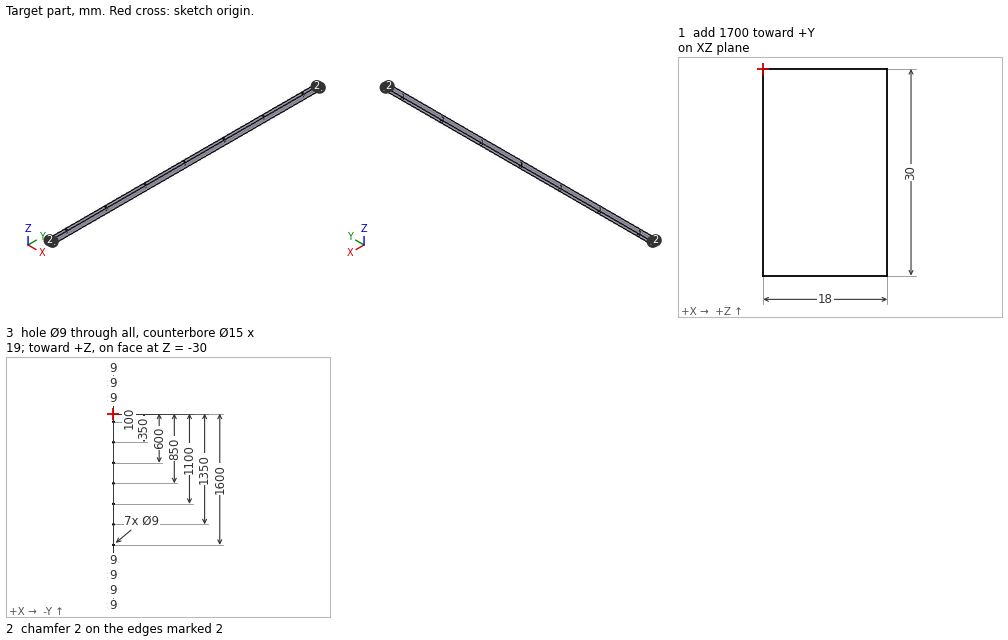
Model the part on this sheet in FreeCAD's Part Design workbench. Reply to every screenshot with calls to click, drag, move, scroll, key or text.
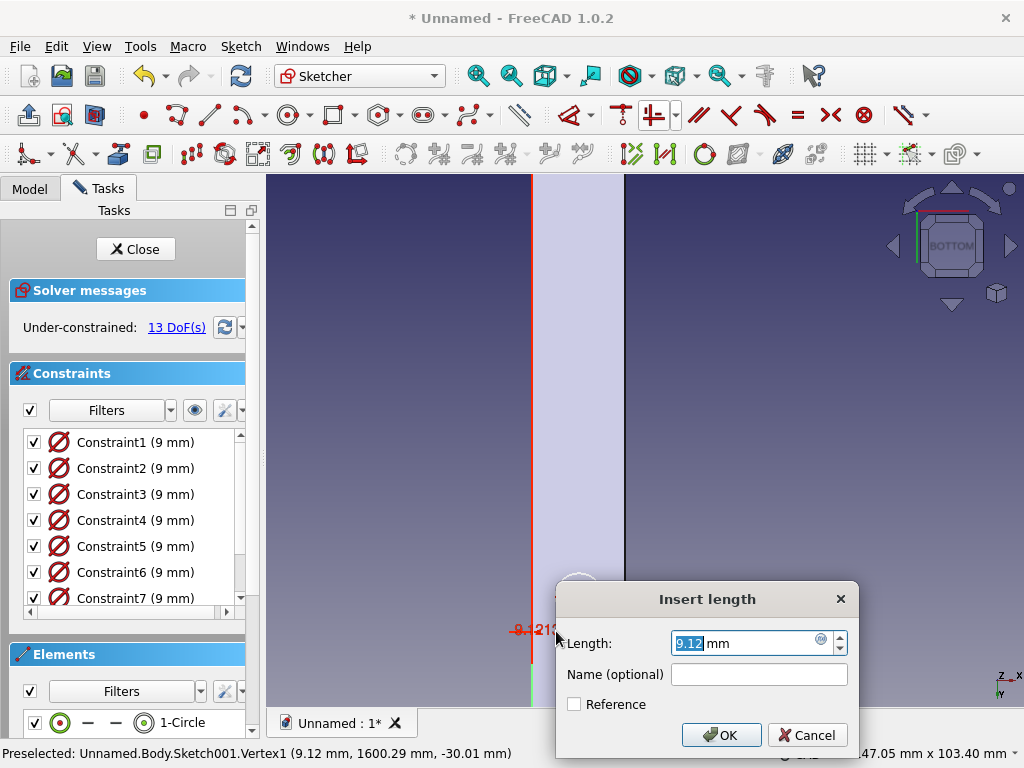
text(9)
key(Return)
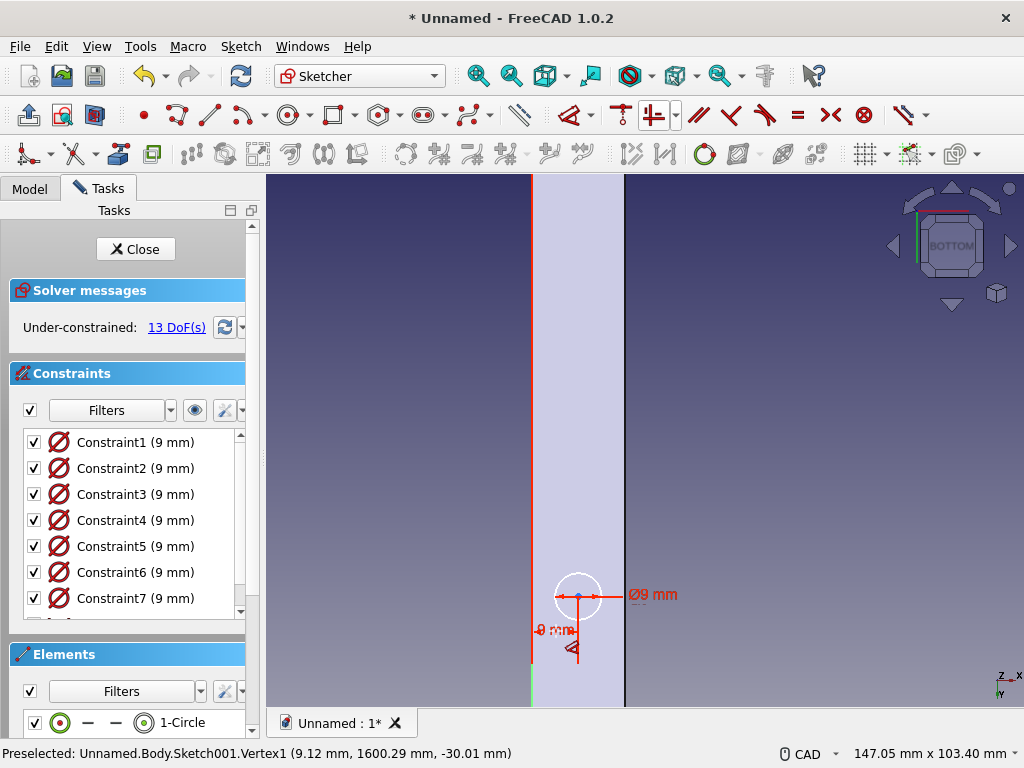
scroll(577, 648, down, 15)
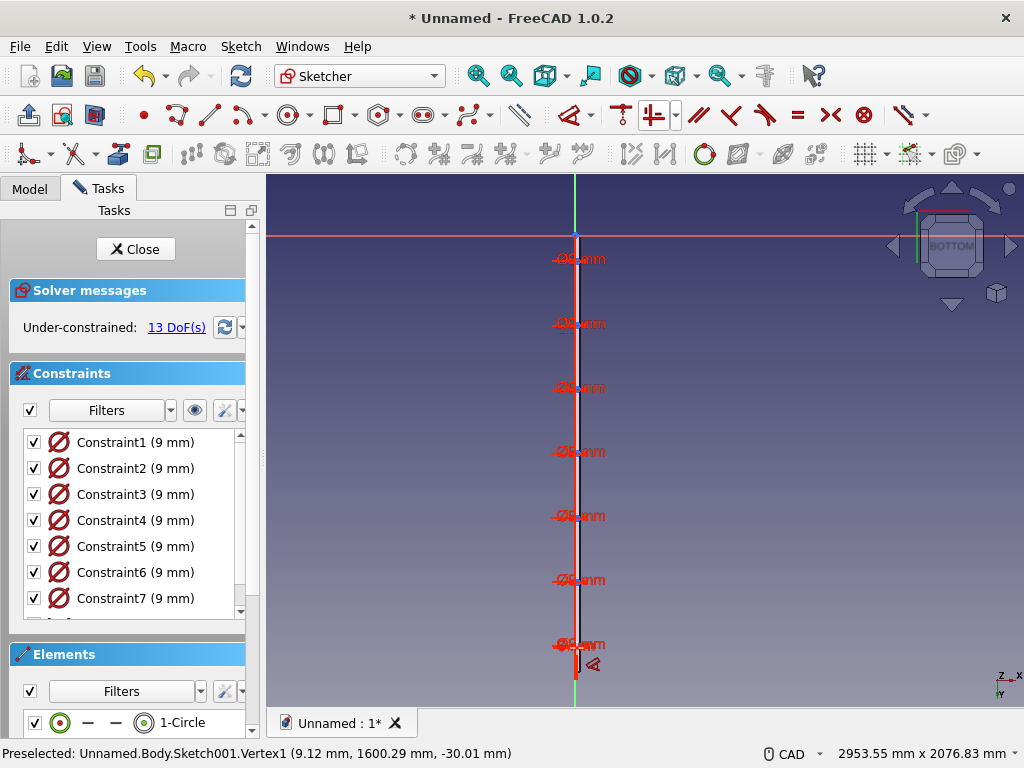
scroll(577, 582, up, 15)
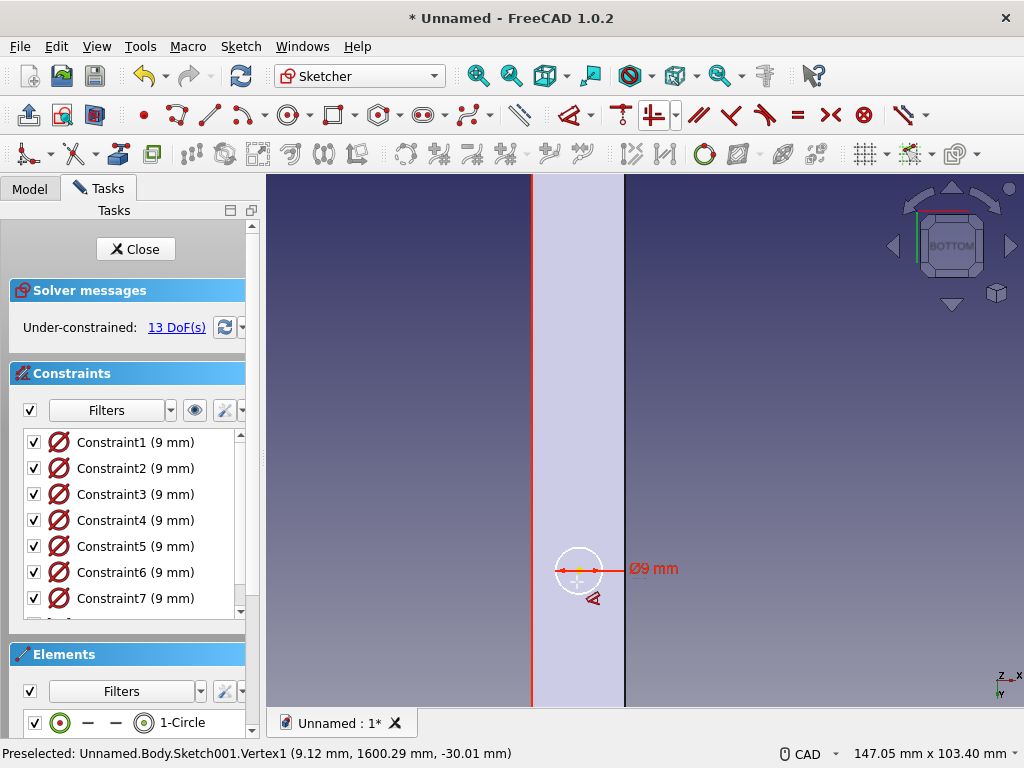
click(579, 571)
click(556, 605)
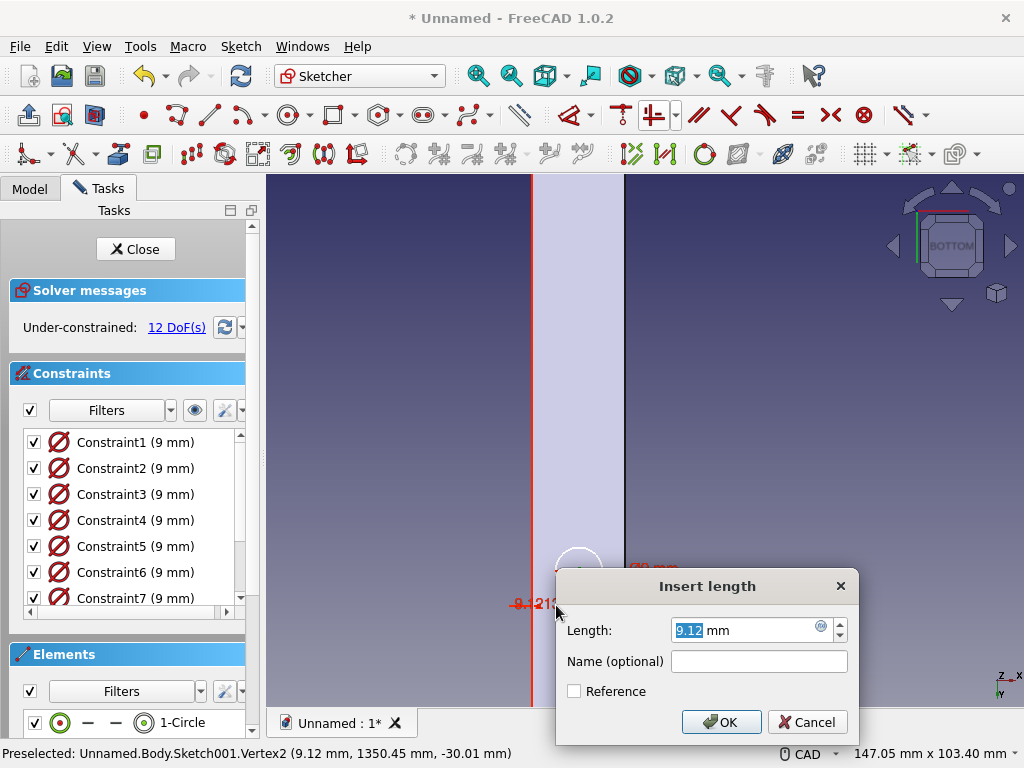
text(9)
key(Return)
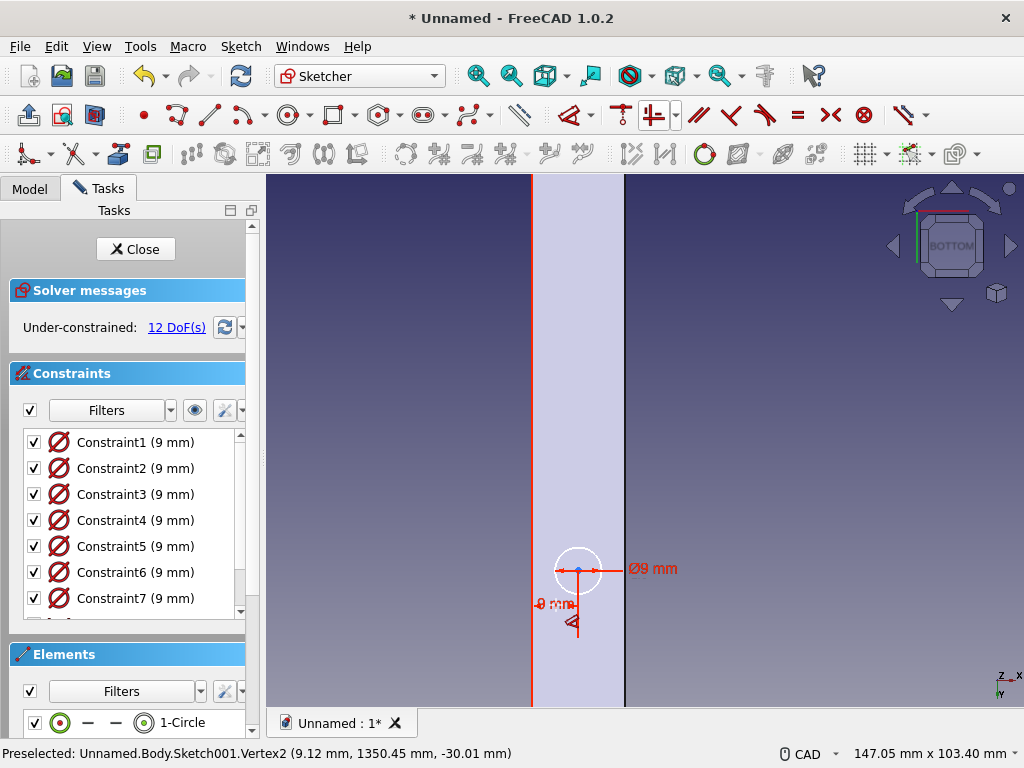
scroll(577, 582, down, 15)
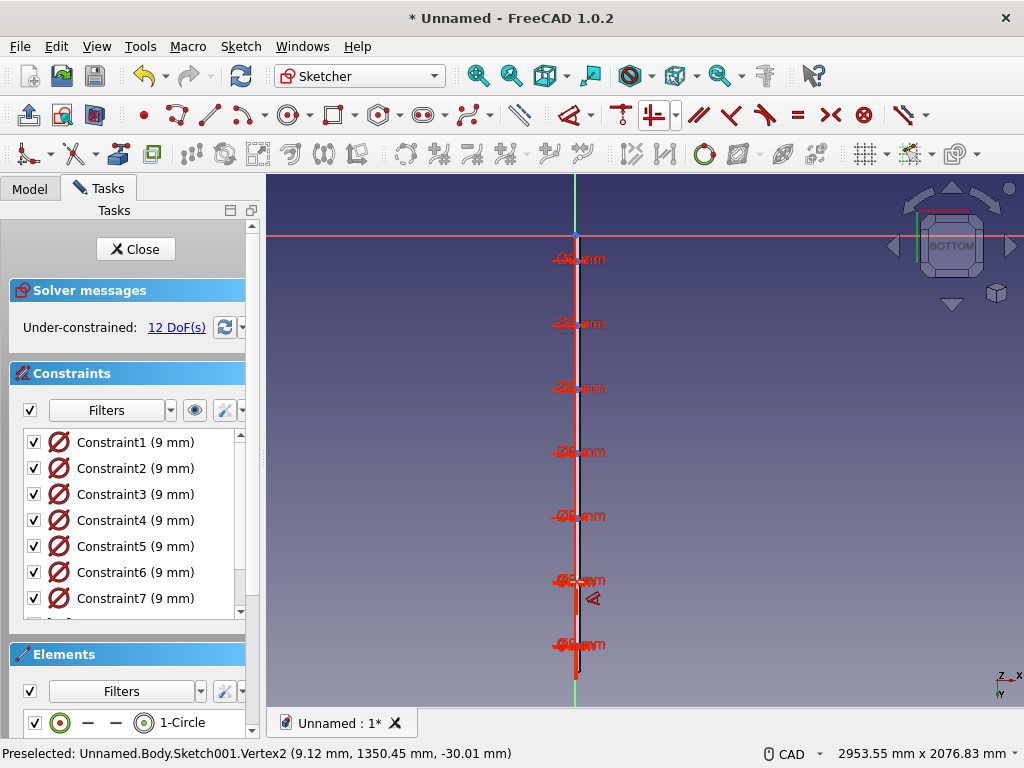
scroll(577, 518, up, 15)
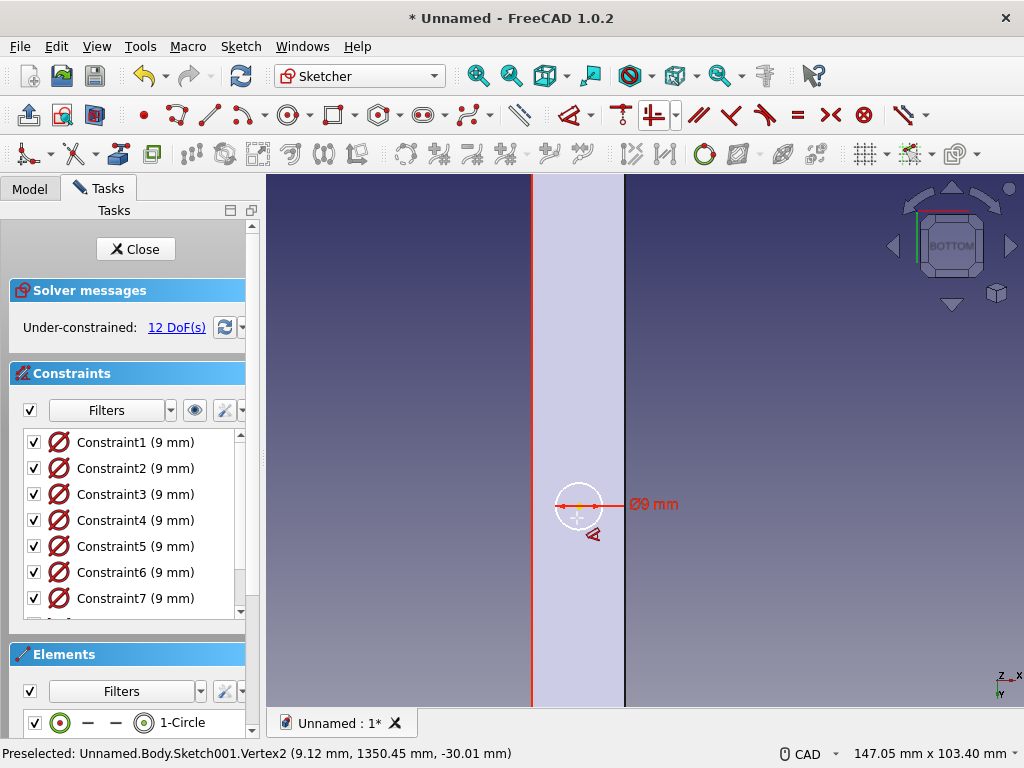
click(579, 506)
click(556, 540)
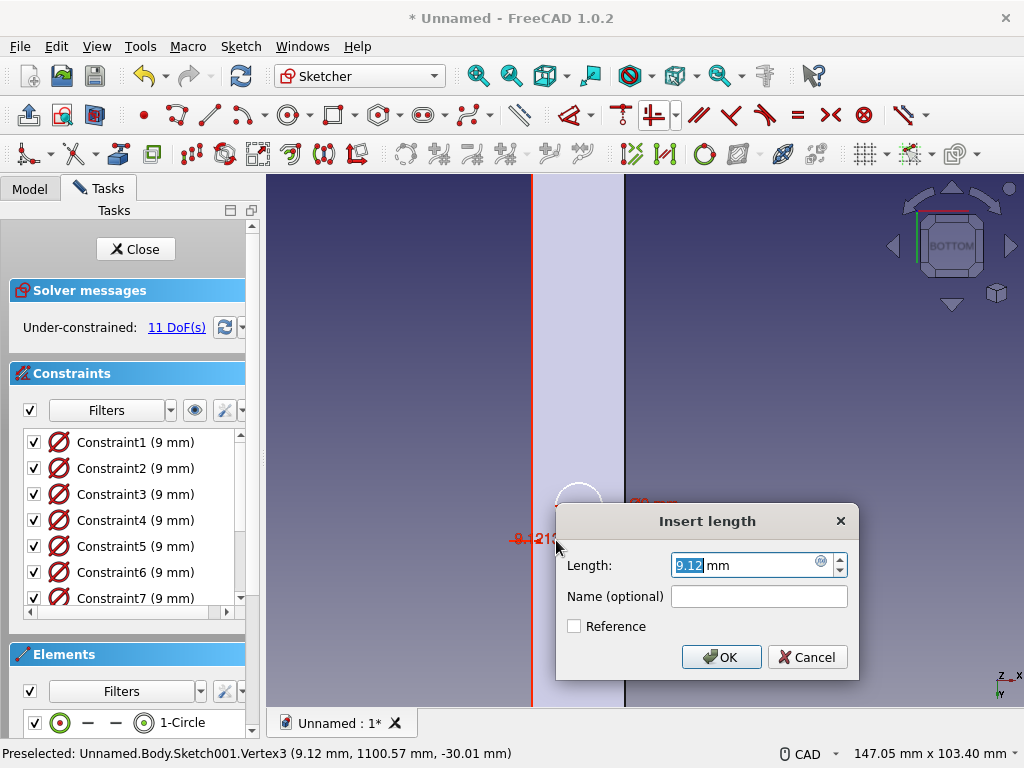
text(9)
key(Return)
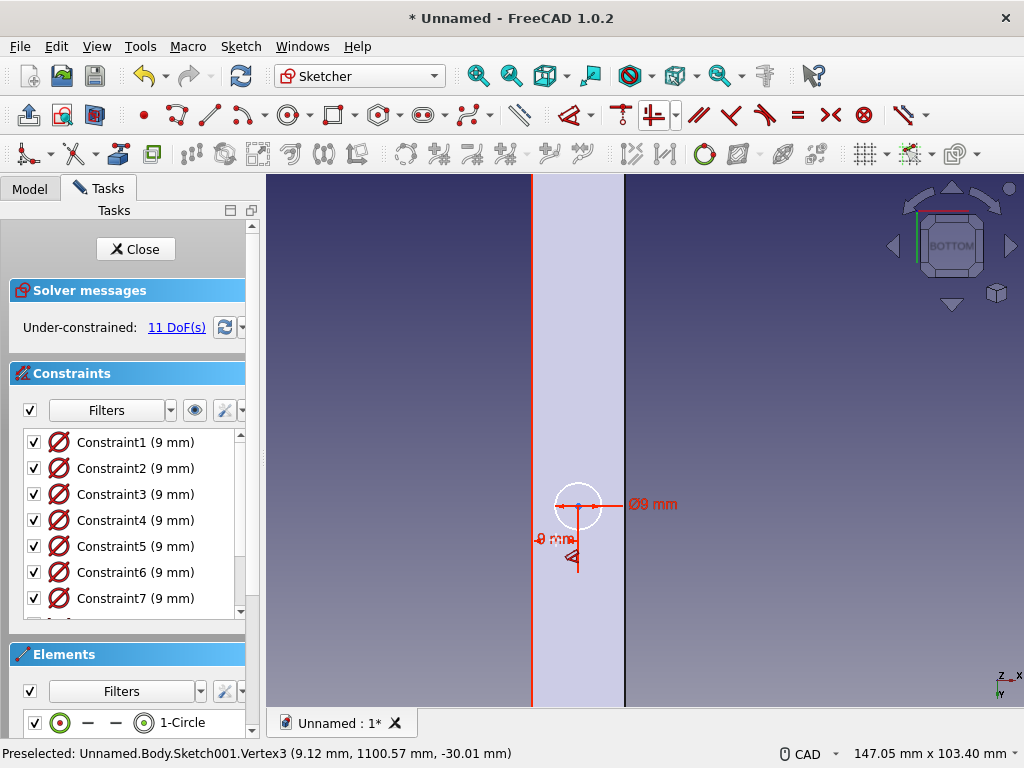
scroll(577, 518, down, 15)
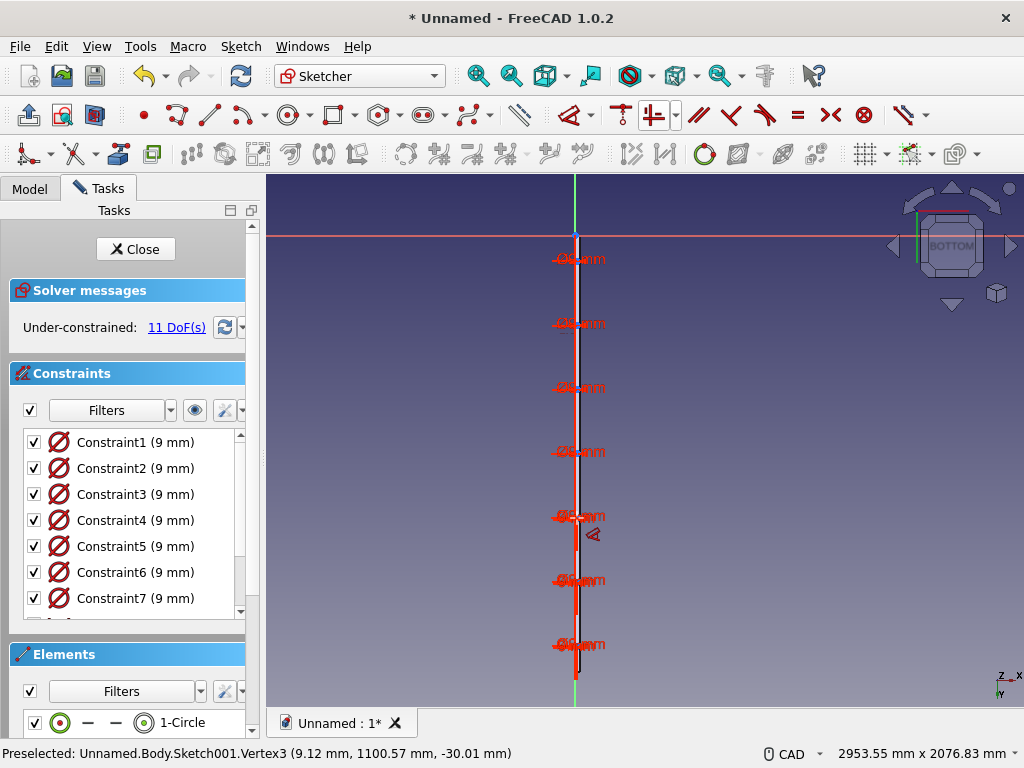
scroll(577, 390, up, 15)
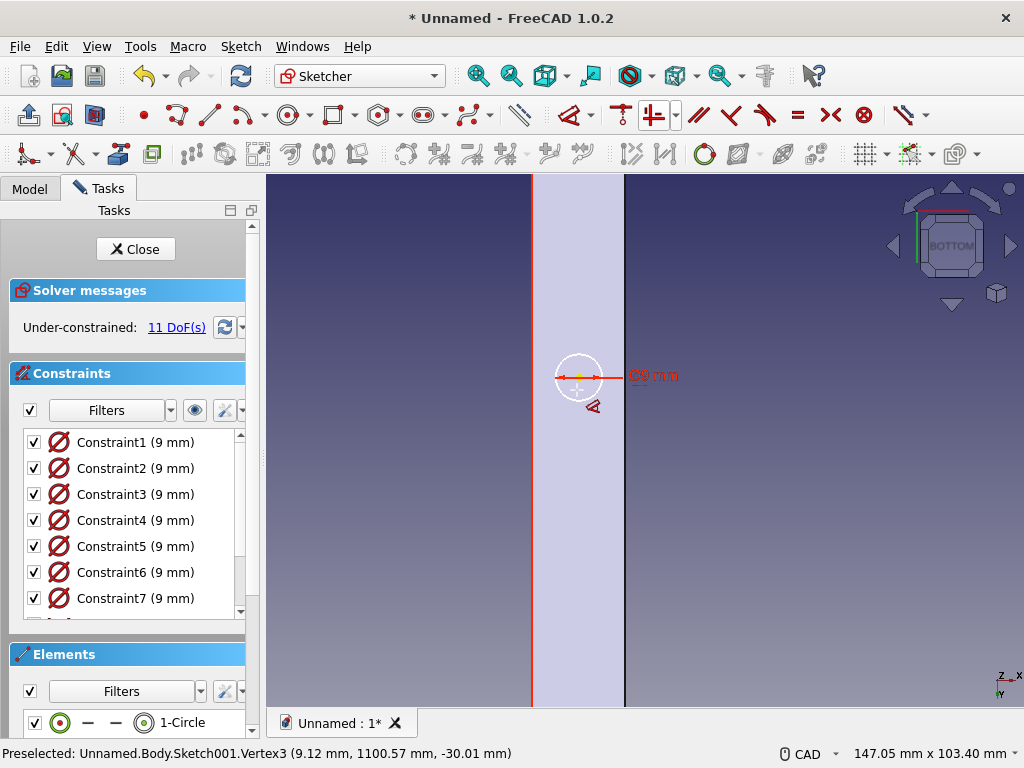
click(579, 378)
click(556, 412)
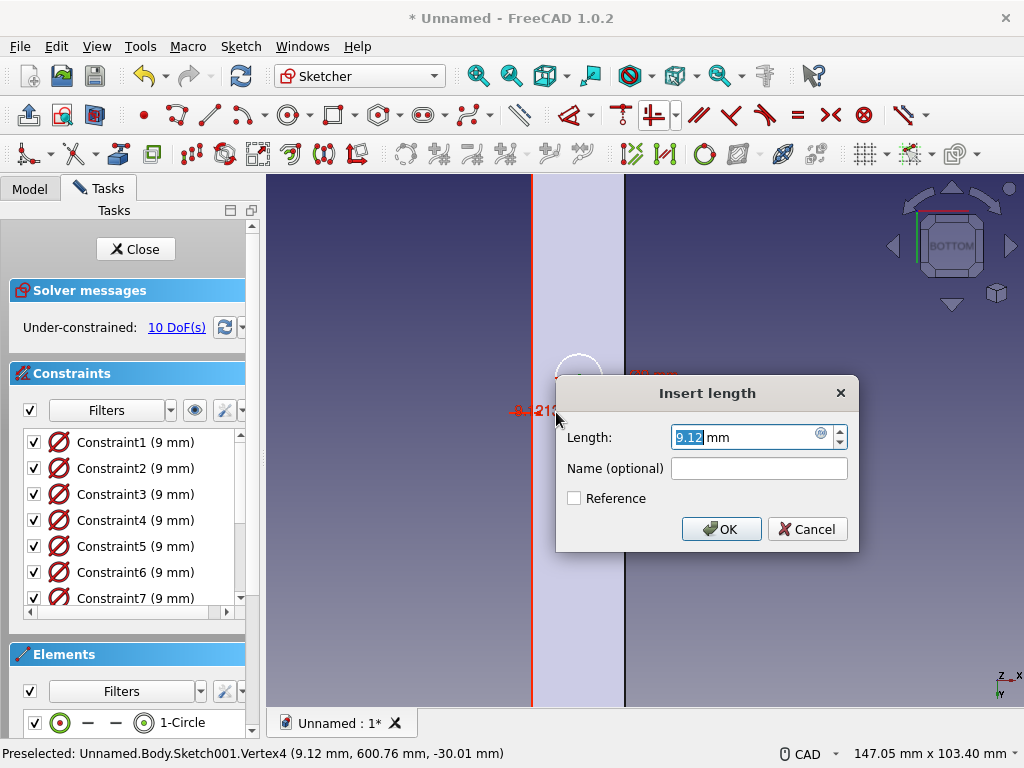
text(9)
key(Return)